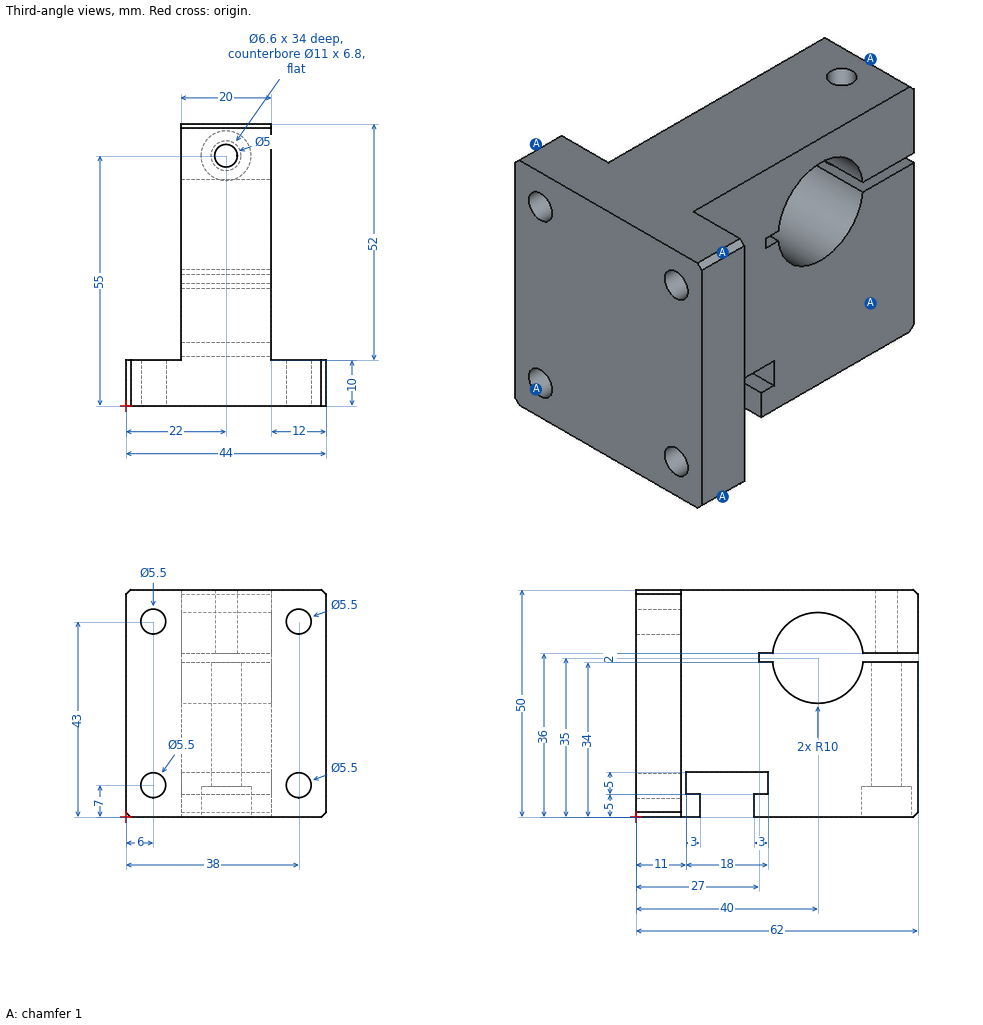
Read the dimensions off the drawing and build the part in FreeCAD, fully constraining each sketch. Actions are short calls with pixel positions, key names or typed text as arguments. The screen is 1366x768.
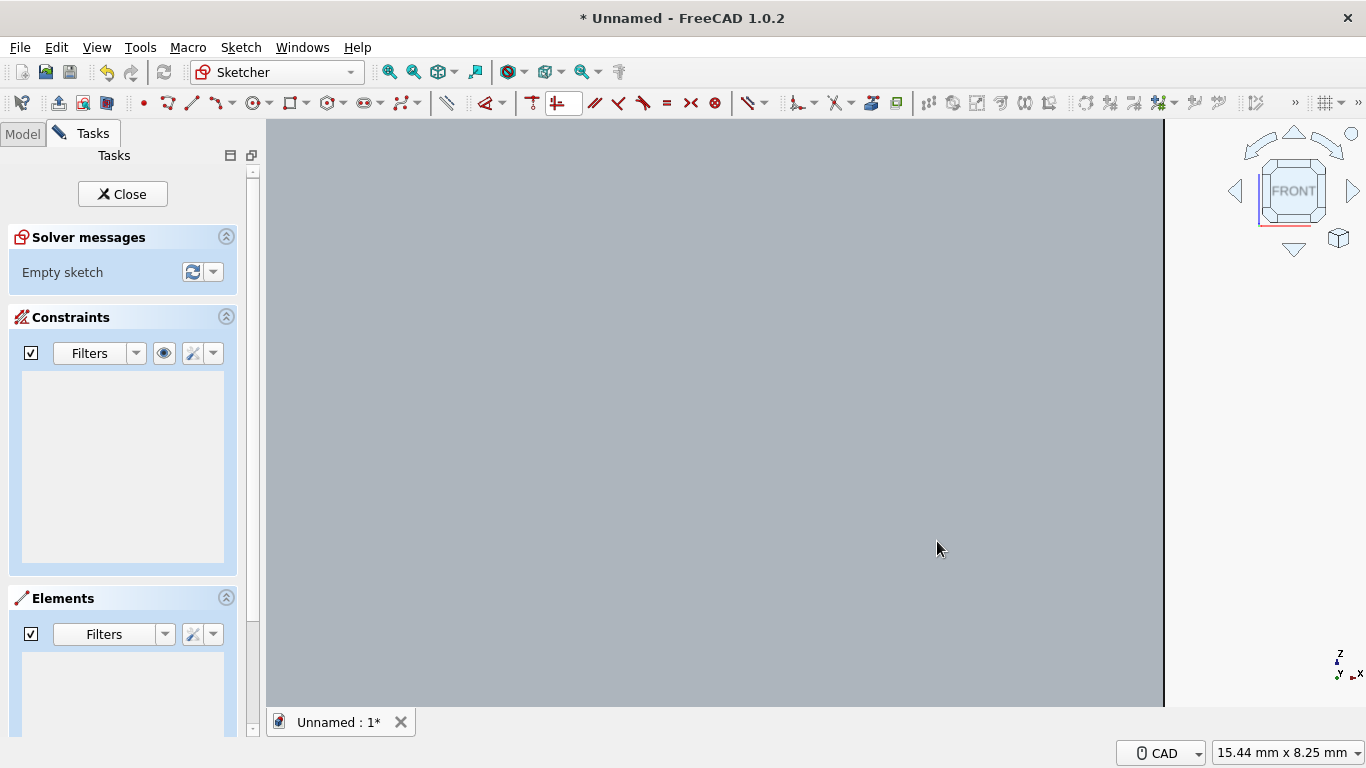
click(254, 104)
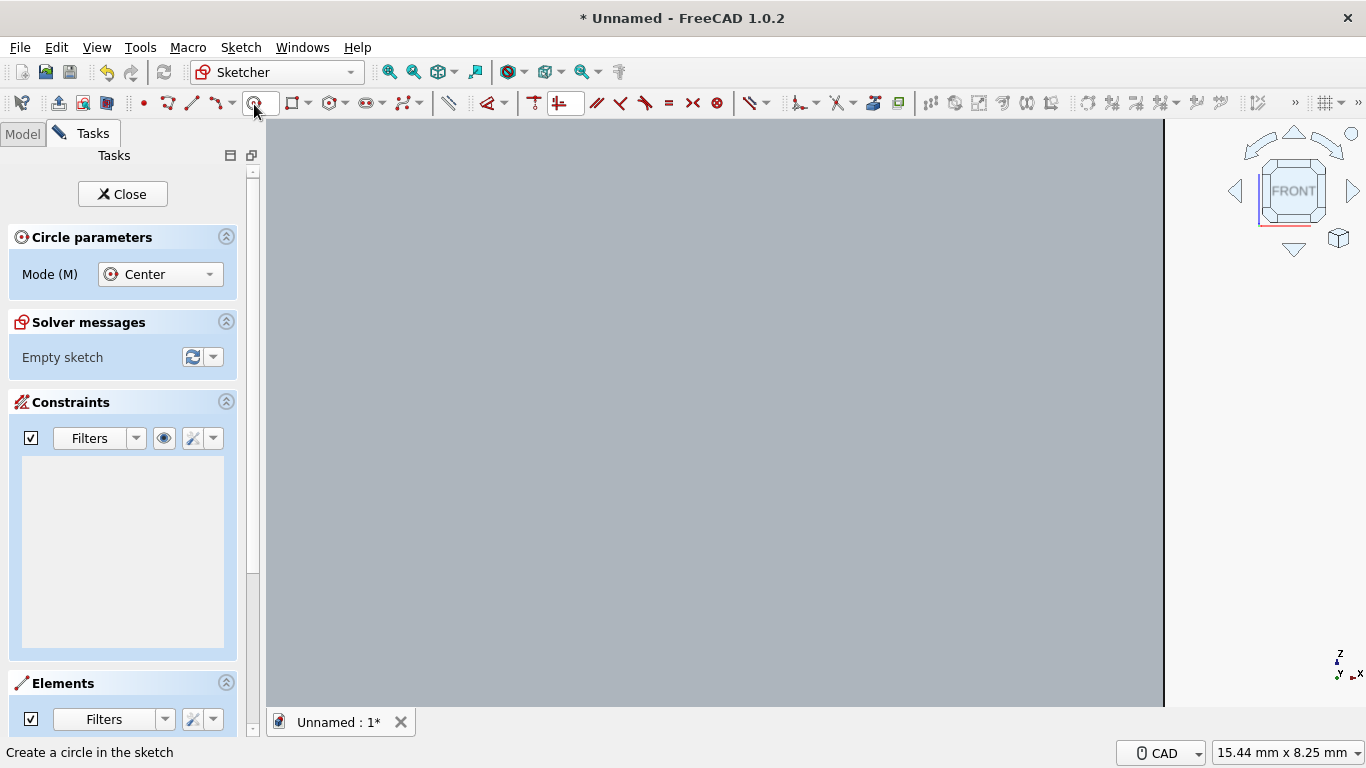
click(737, 405)
move(875, 266)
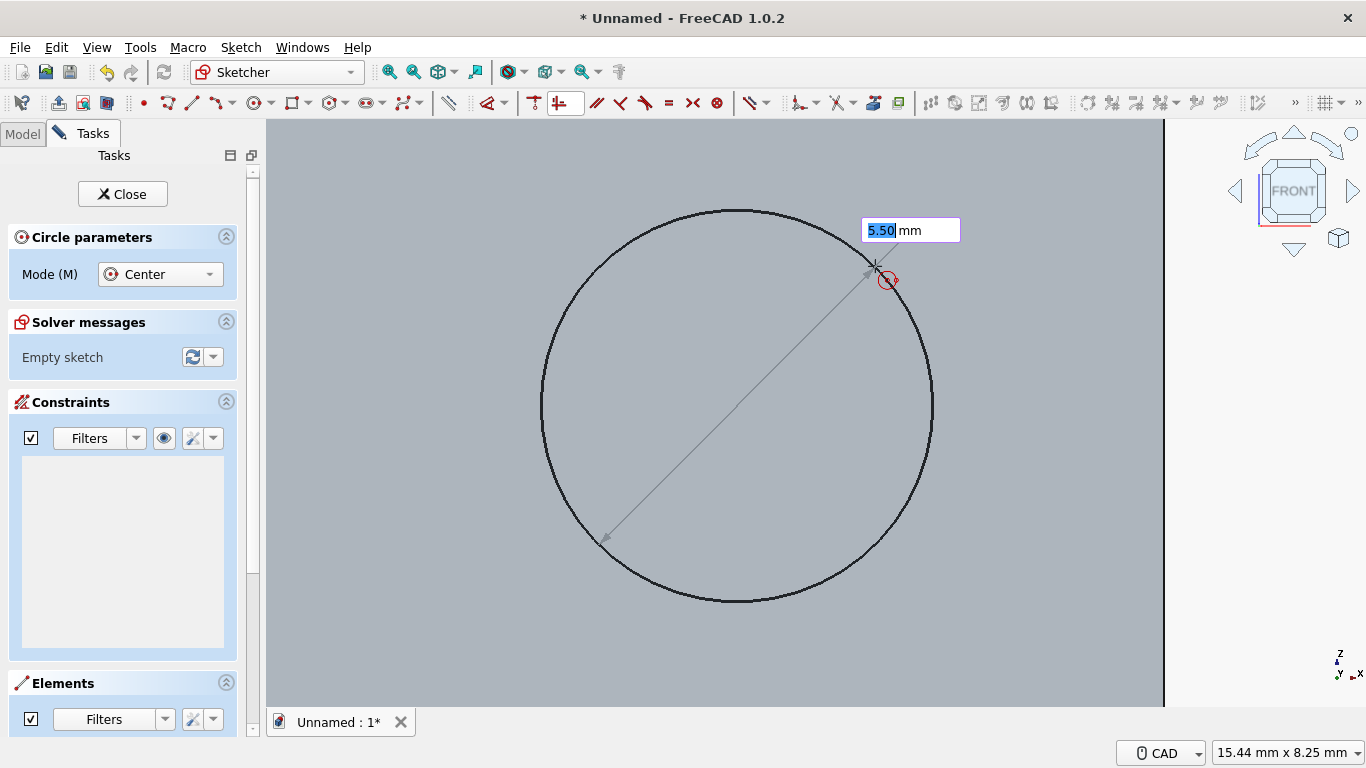
text(5.5)
key(Return)
key(Escape)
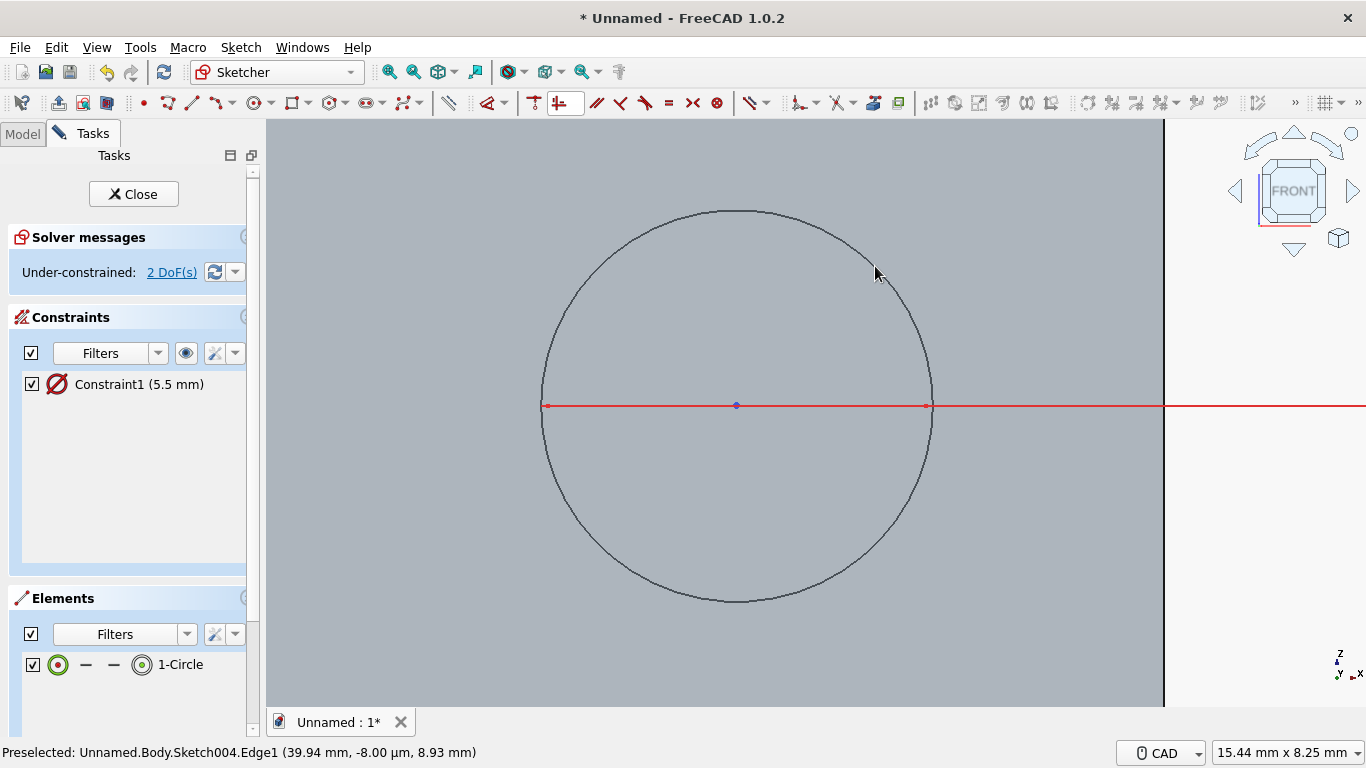
click(488, 104)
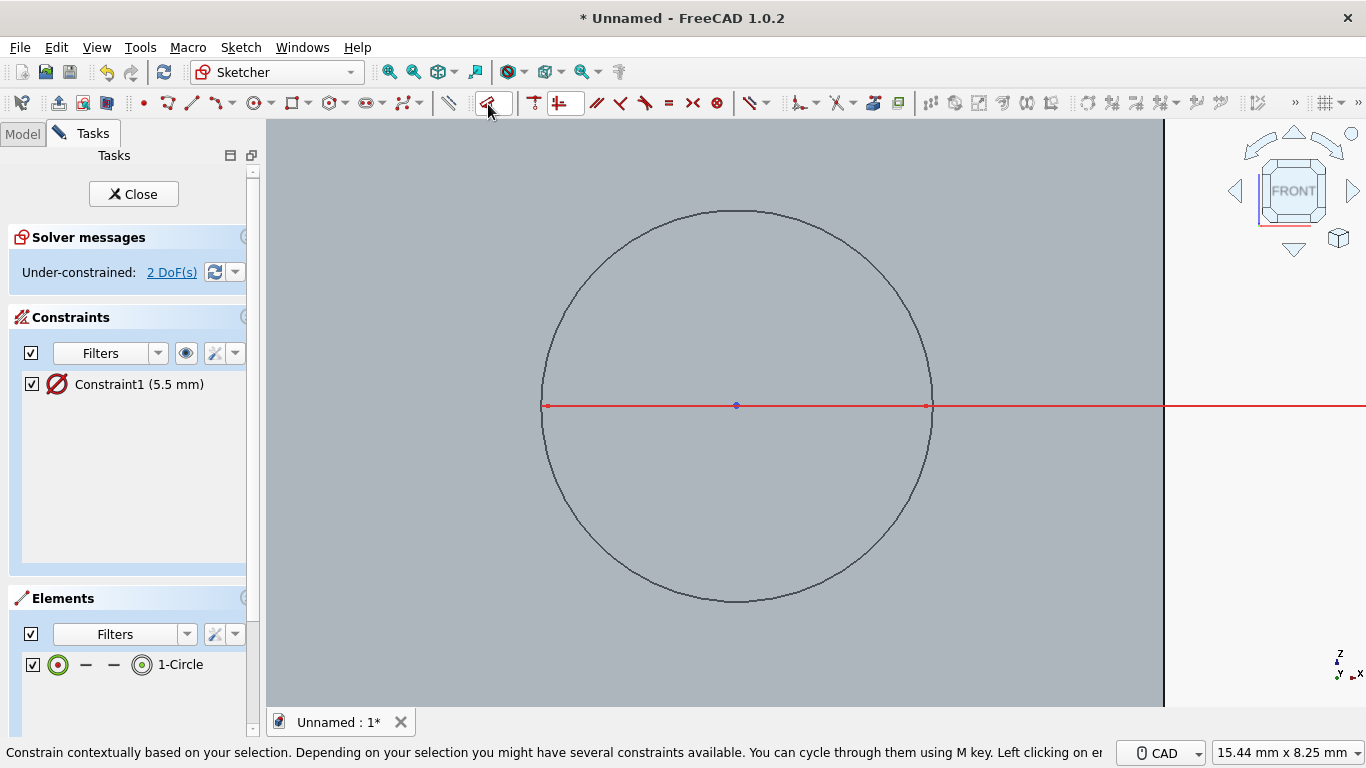
click(737, 406)
click(771, 542)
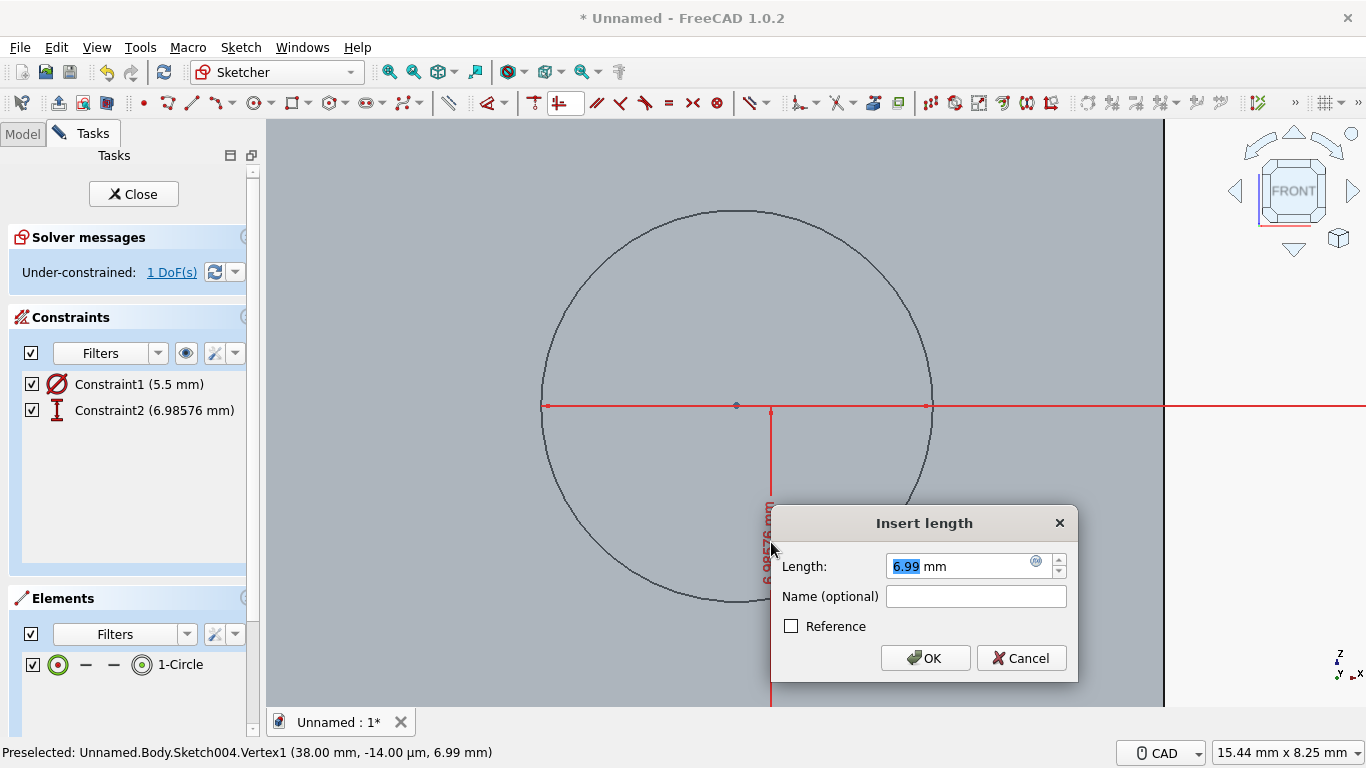
text(7)
key(Return)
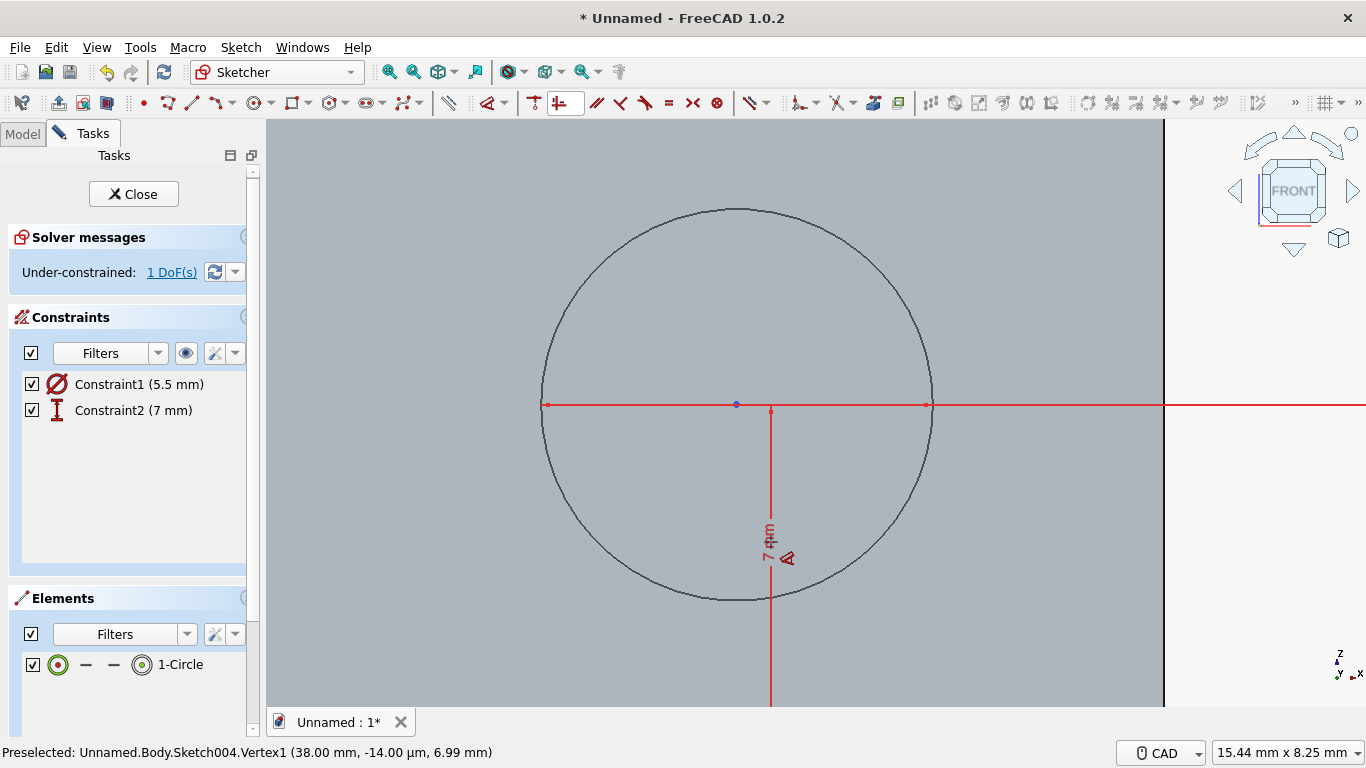
click(737, 405)
click(515, 371)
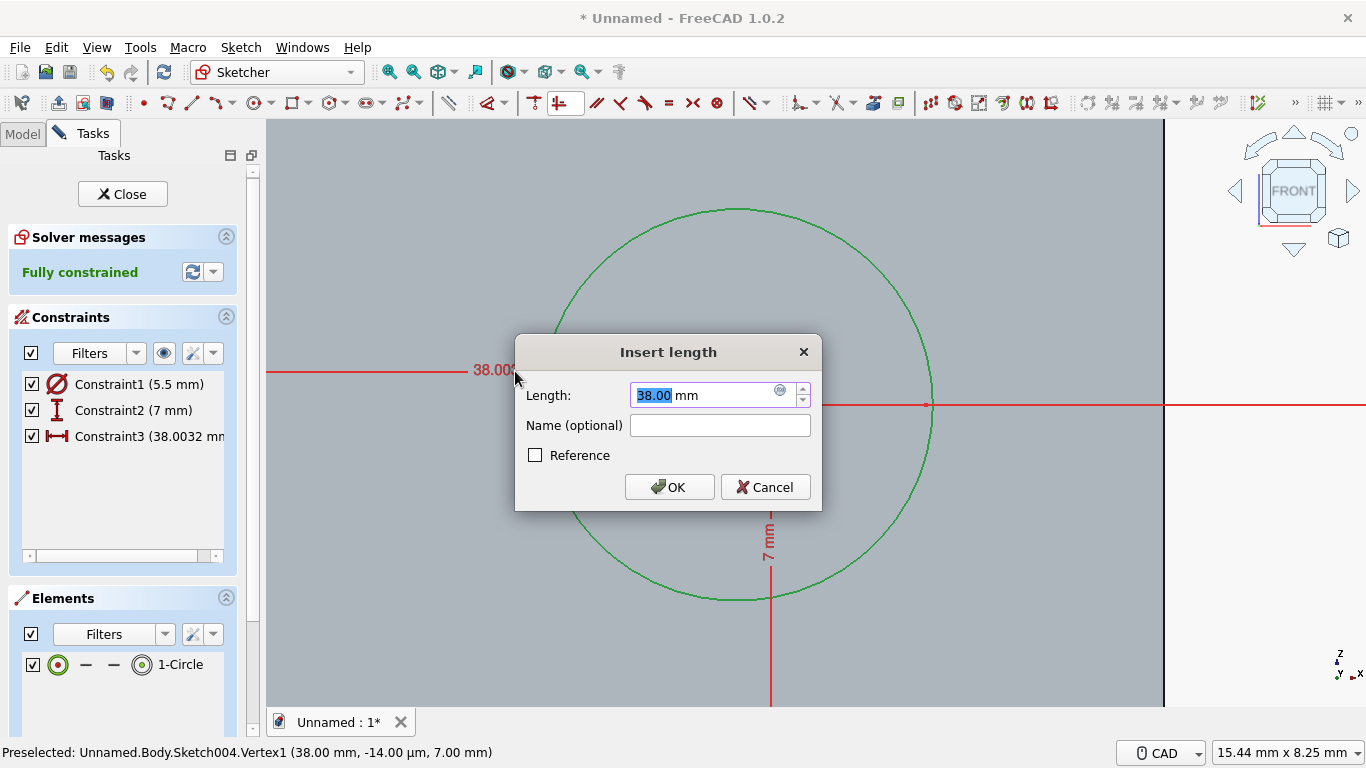
text(38)
key(Return)
key(Escape)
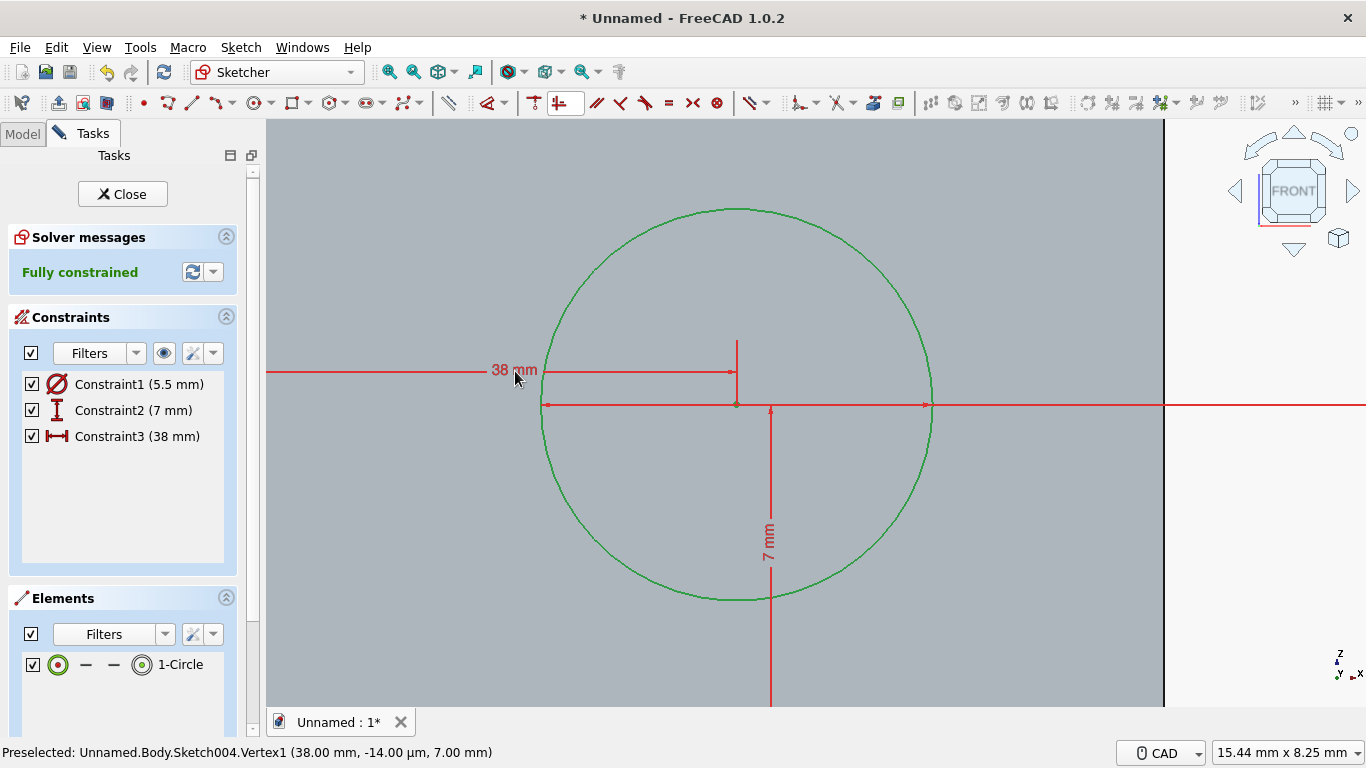
click(123, 194)